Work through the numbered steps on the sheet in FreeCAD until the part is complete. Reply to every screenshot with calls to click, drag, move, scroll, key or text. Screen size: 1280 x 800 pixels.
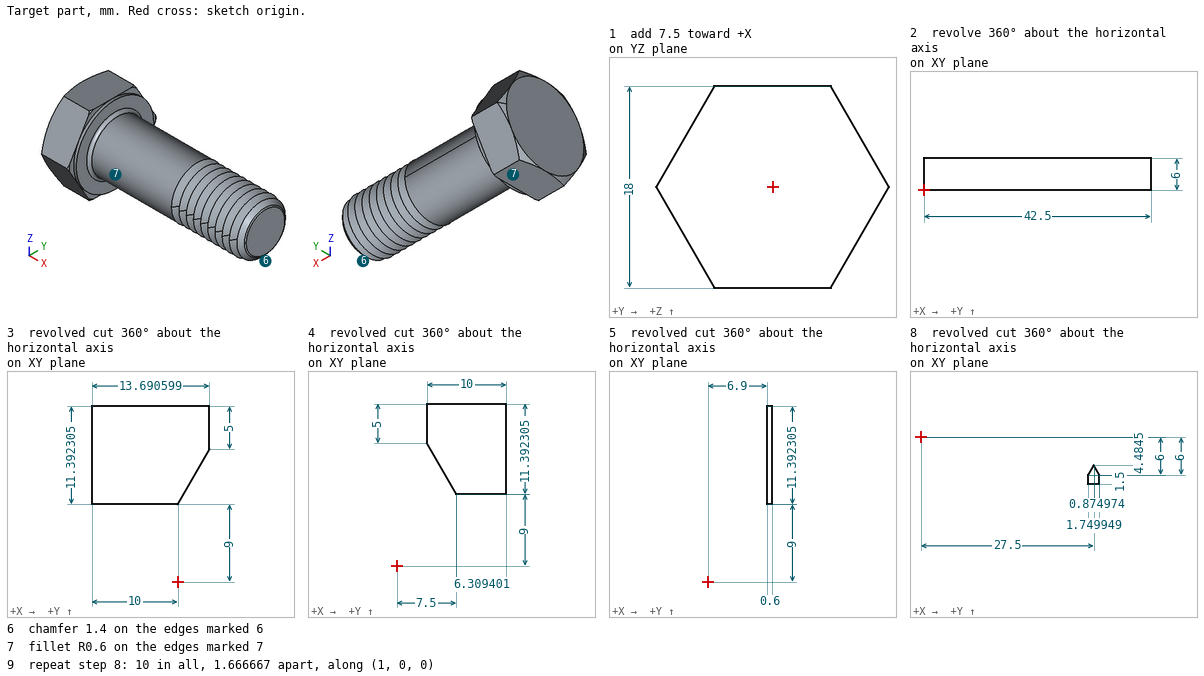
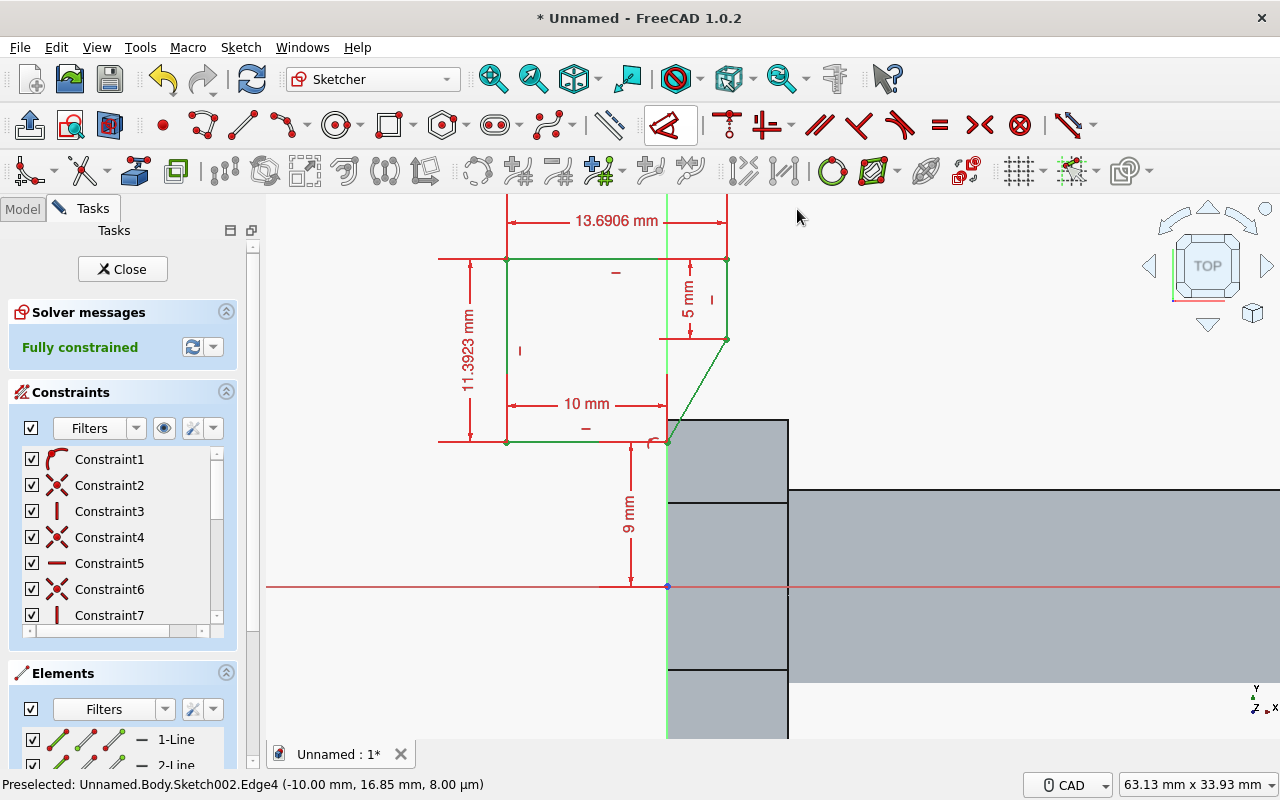
click(123, 269)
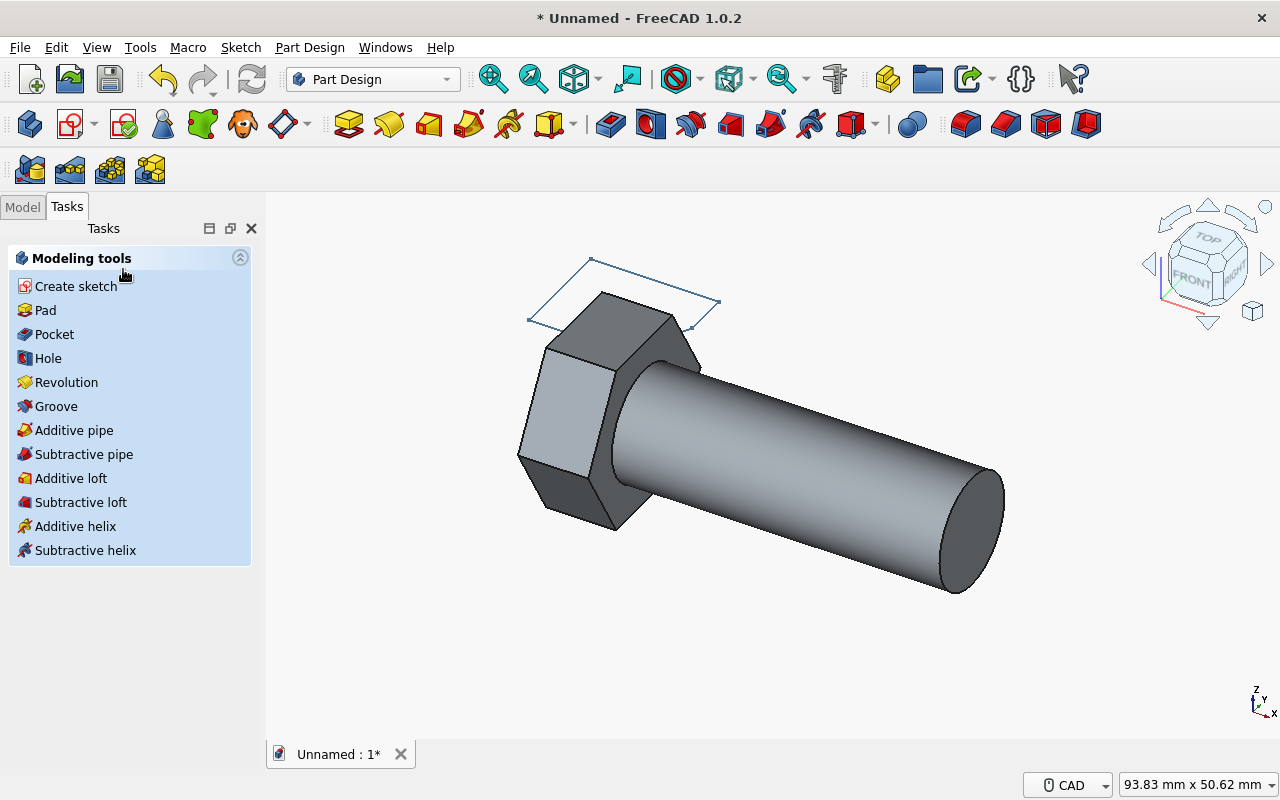
click(692, 124)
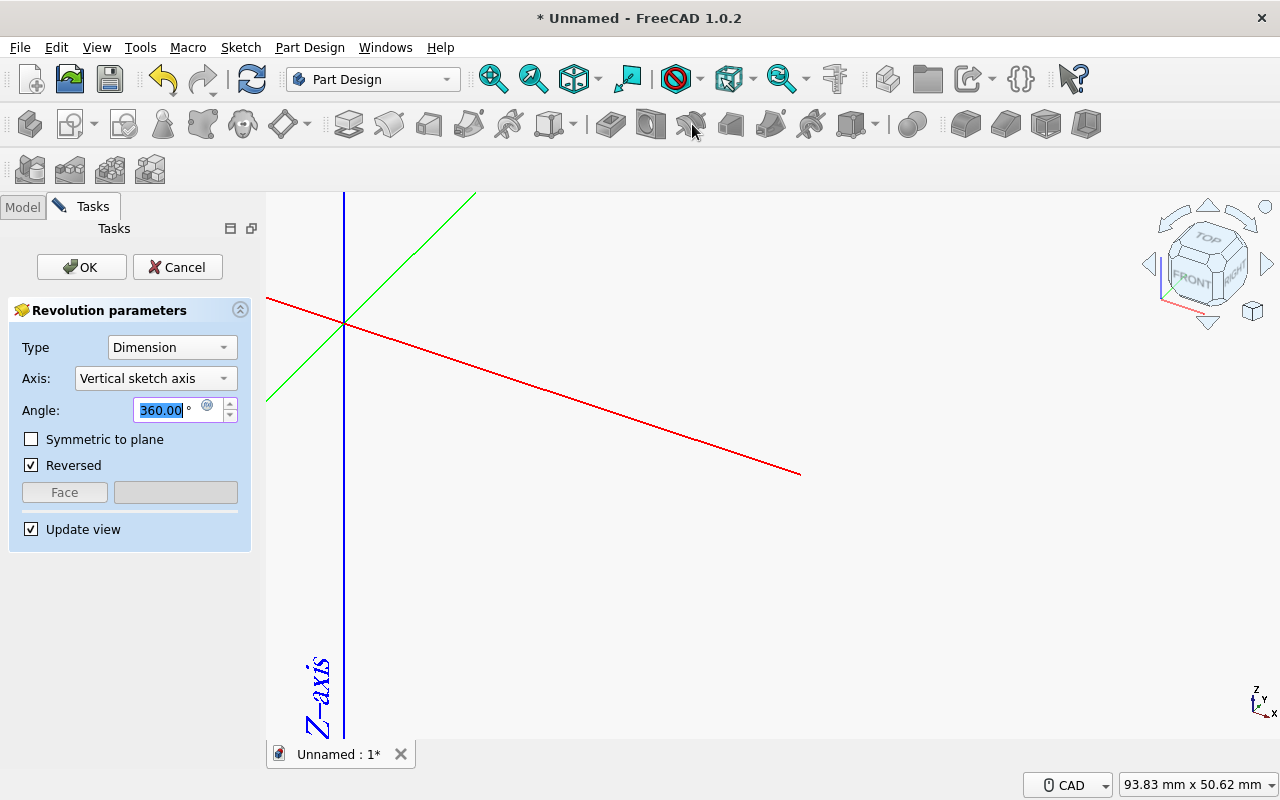
click(156, 378)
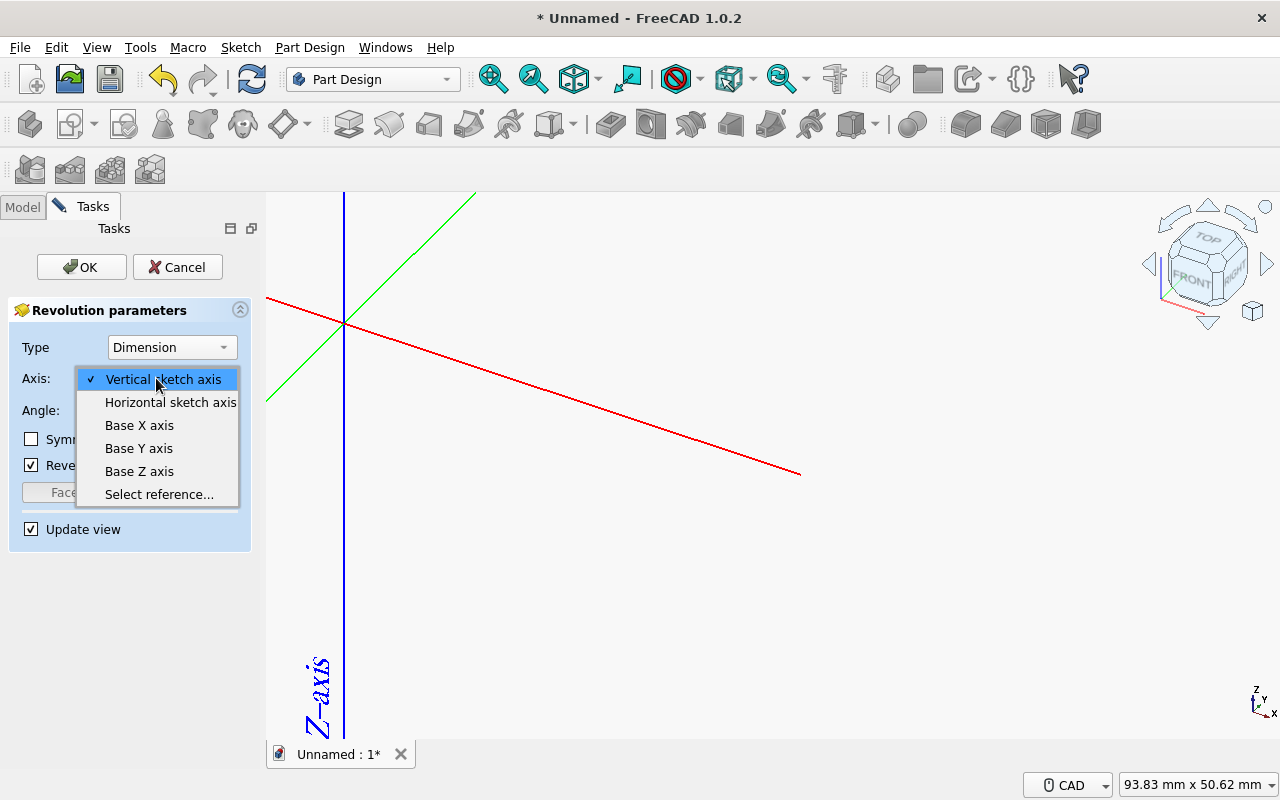
click(156, 402)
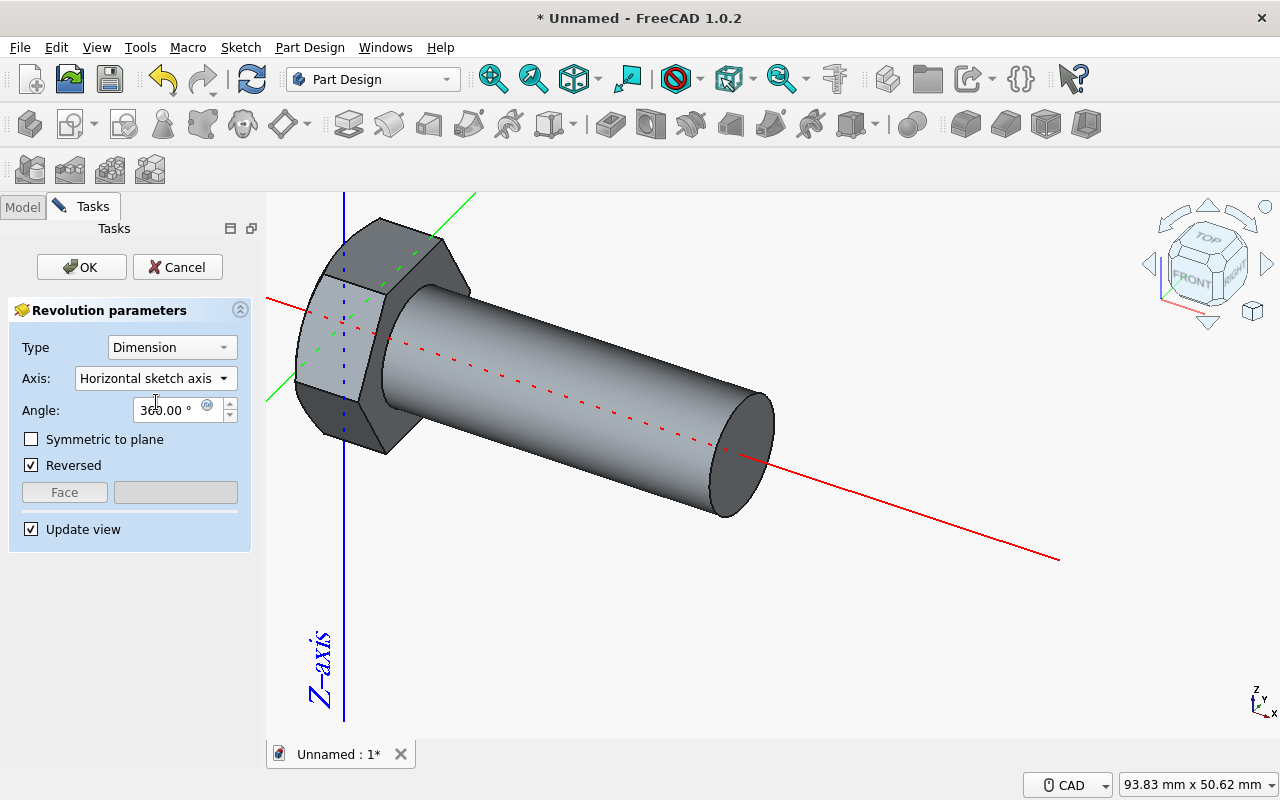
click(82, 267)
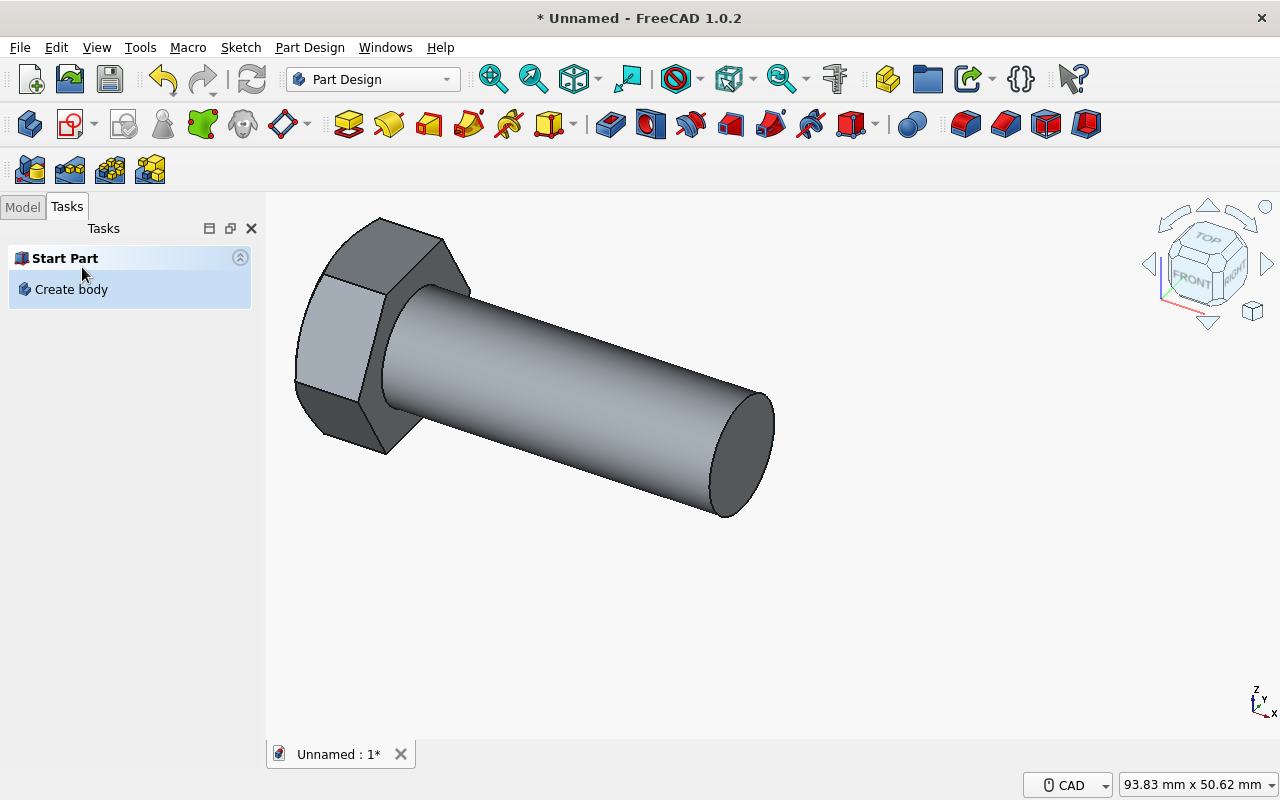
key(v)
key(f)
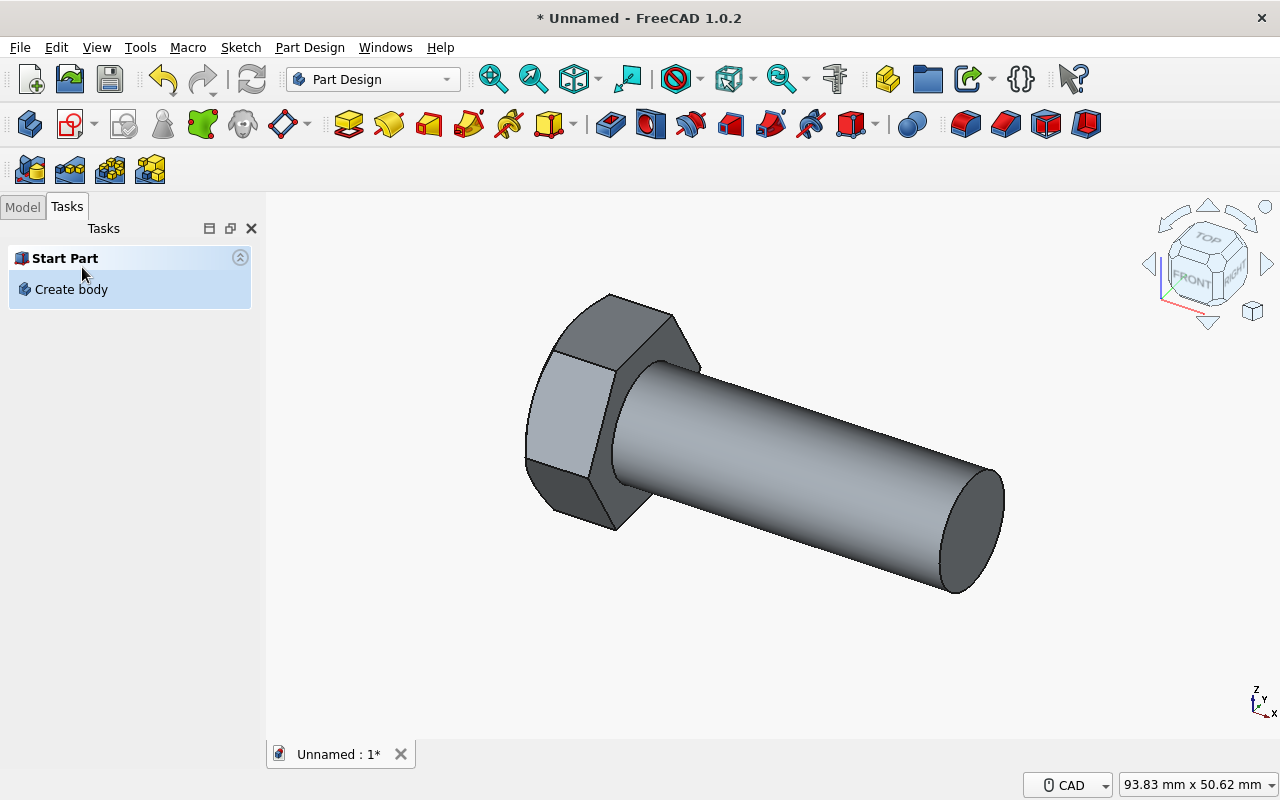
click(70, 124)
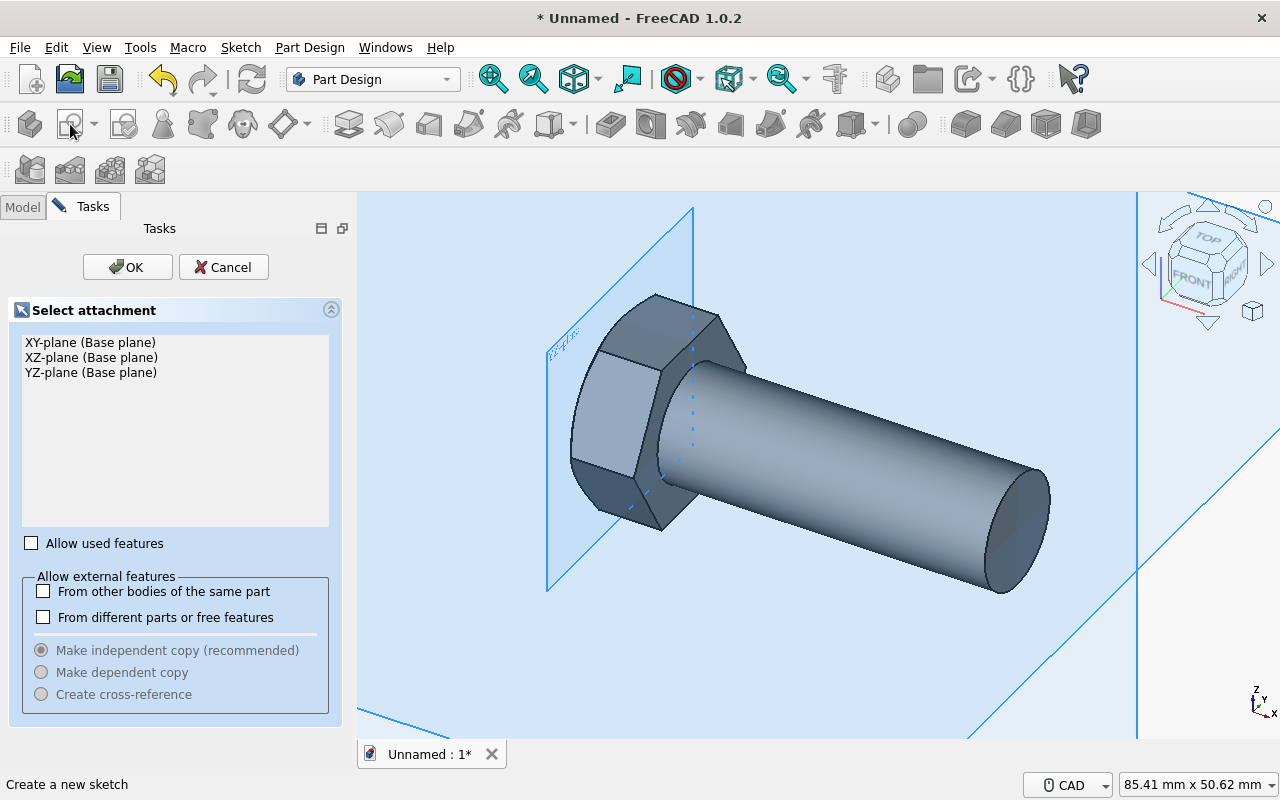
click(82, 342)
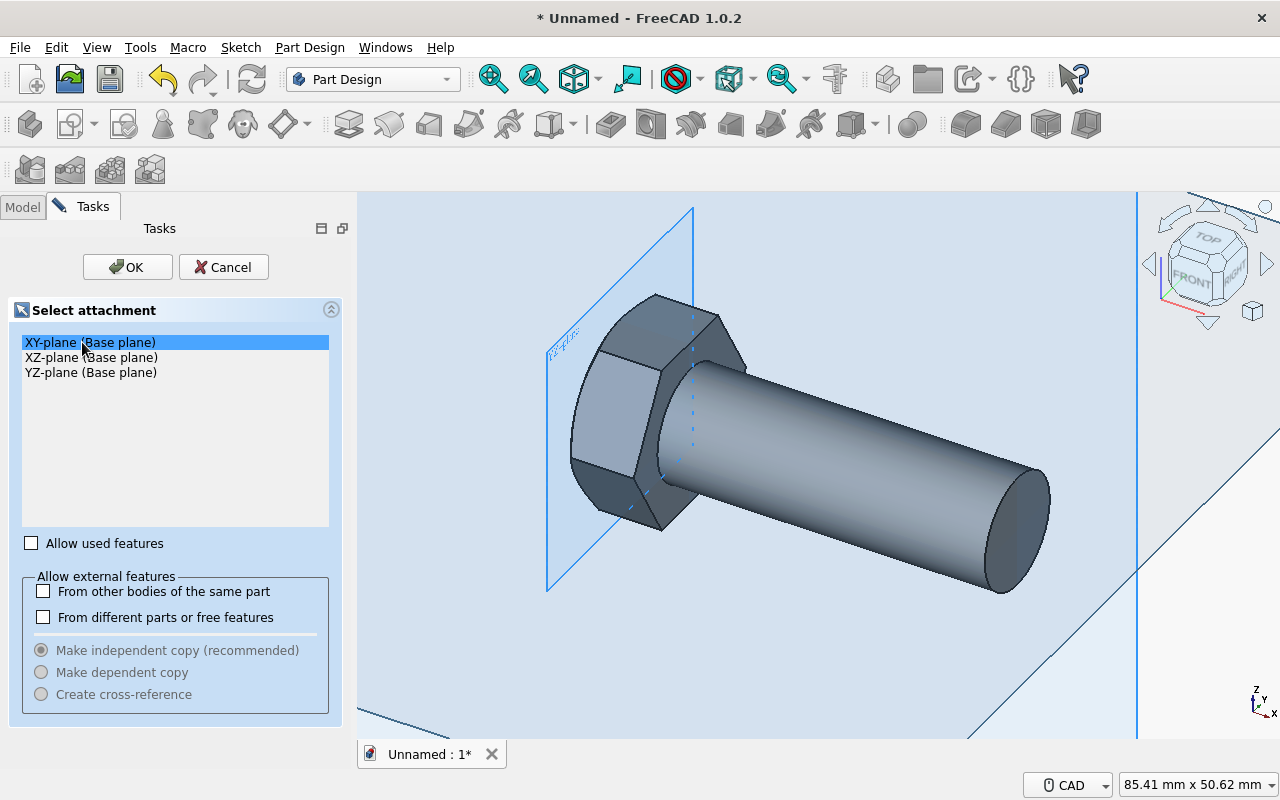
click(128, 267)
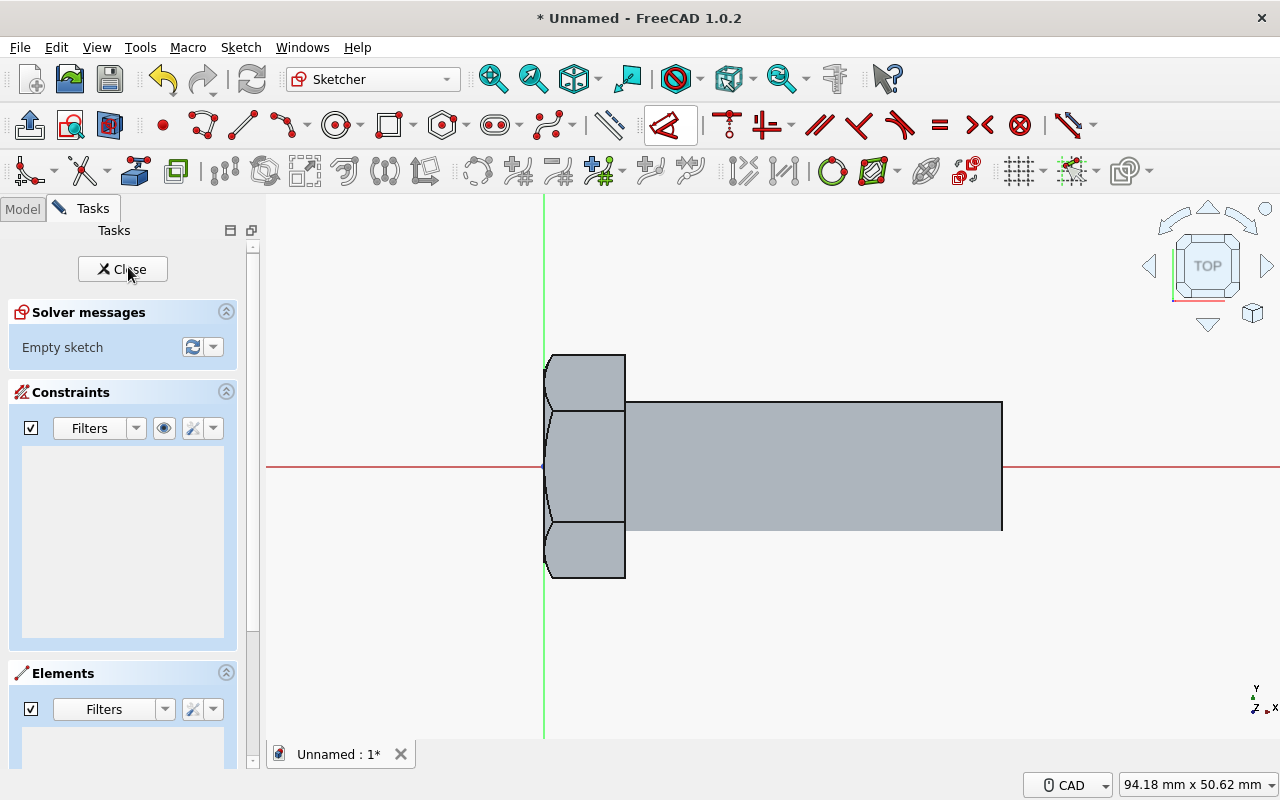
key(q)
key(s)